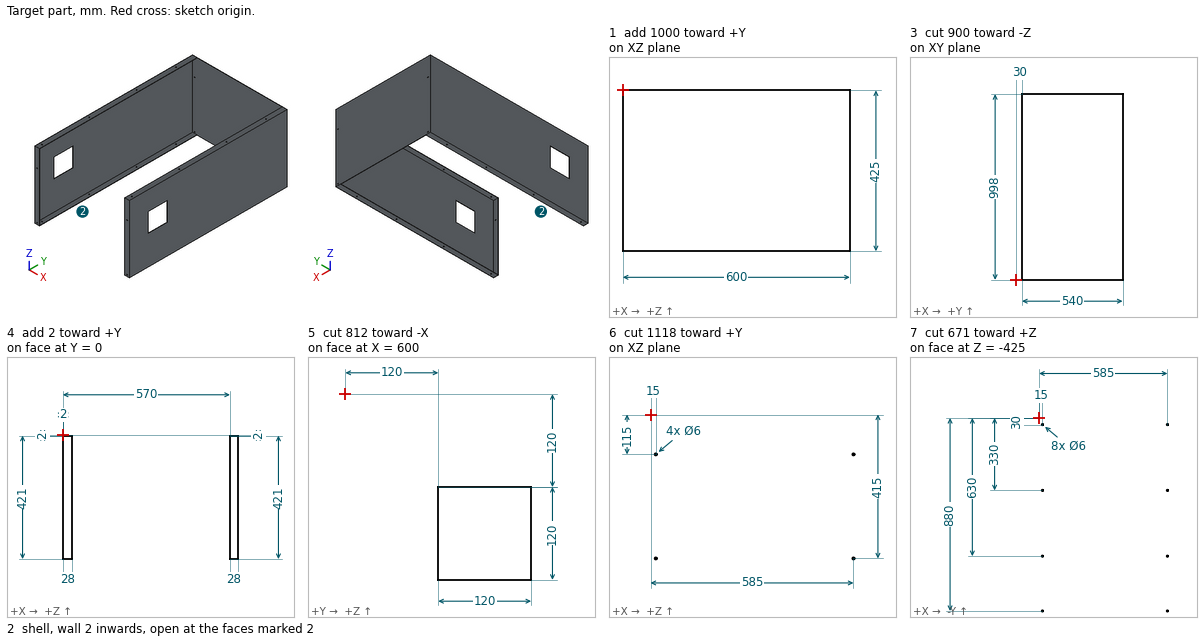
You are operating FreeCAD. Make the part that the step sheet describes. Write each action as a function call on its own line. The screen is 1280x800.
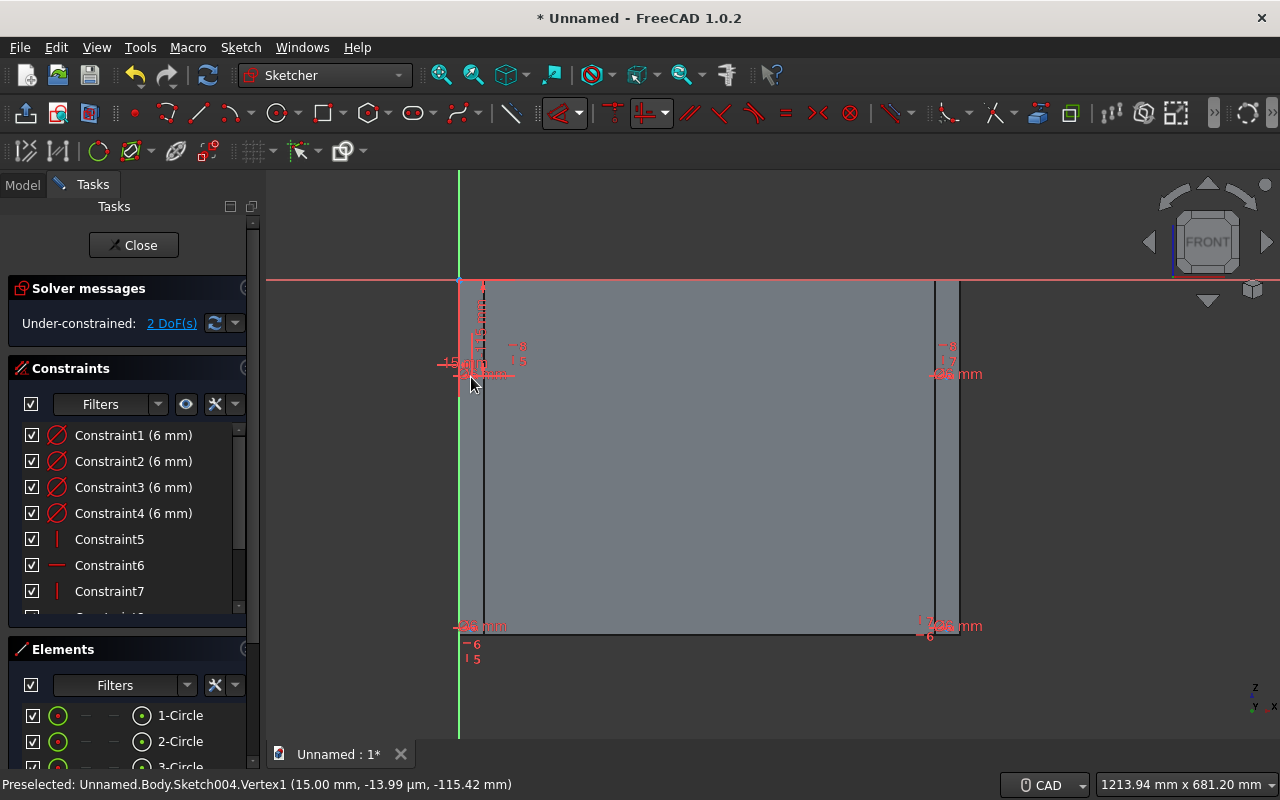
click(947, 628)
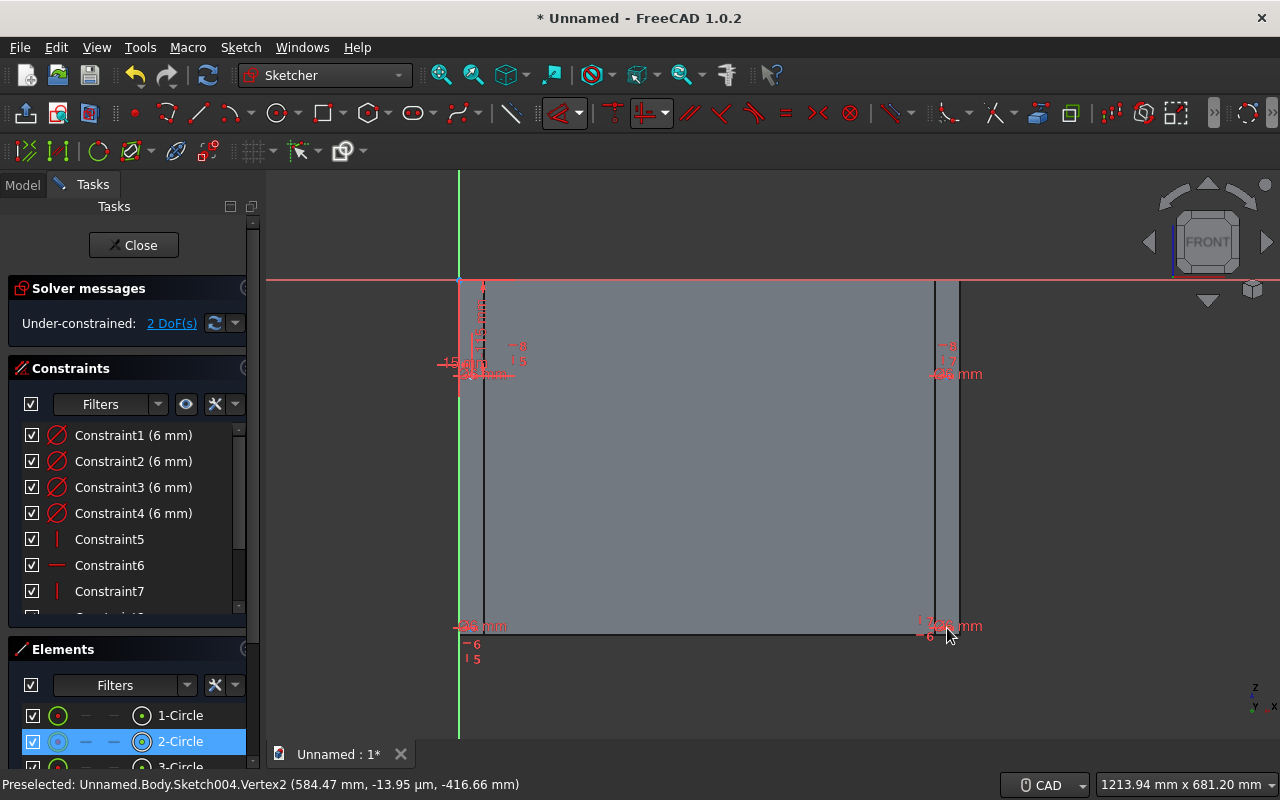
click(582, 114)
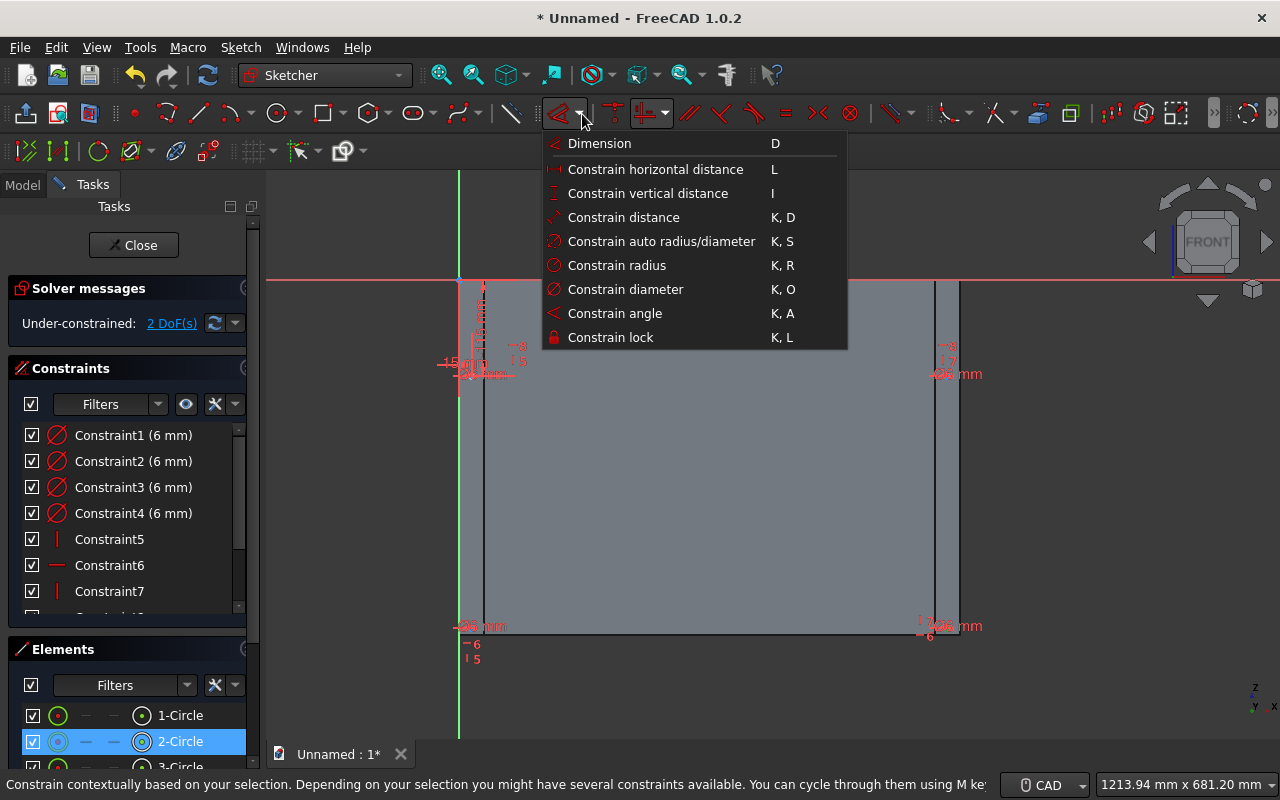
click(695, 169)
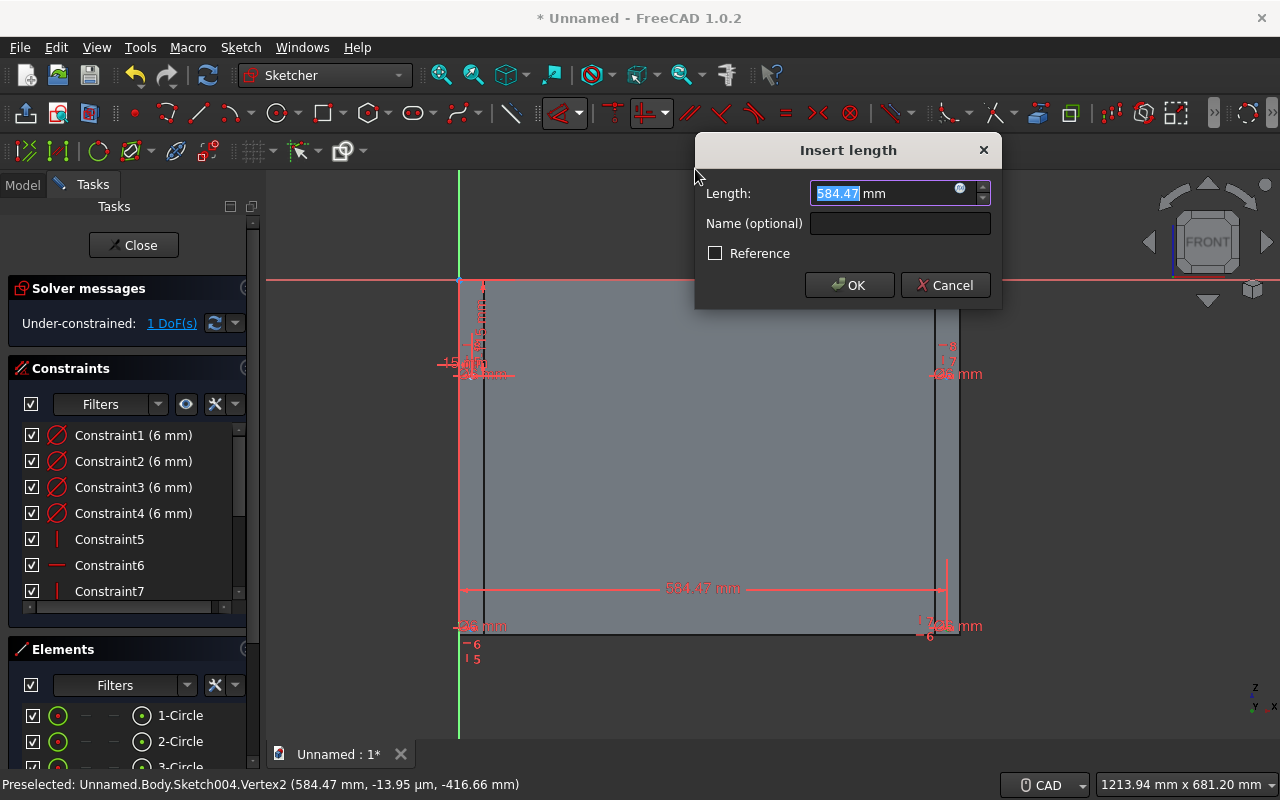
text(585)
key(Return)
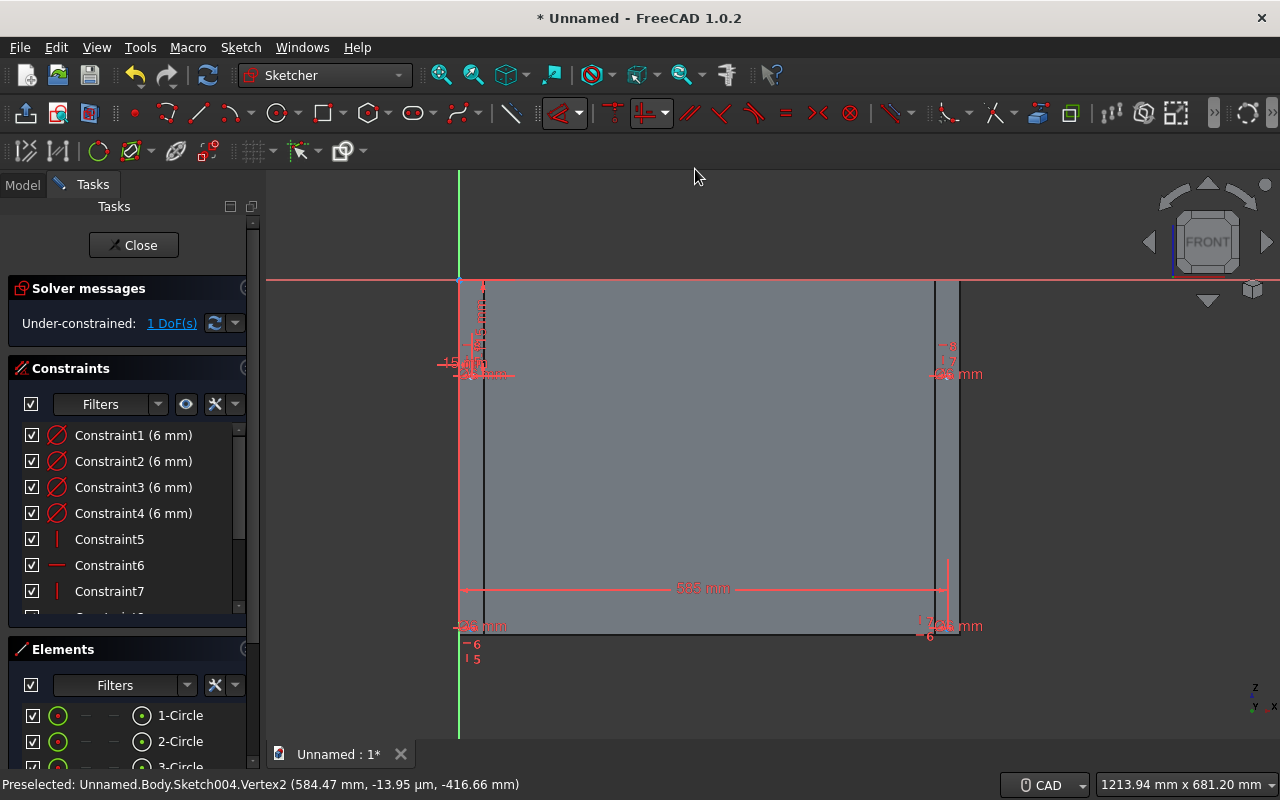
click(948, 628)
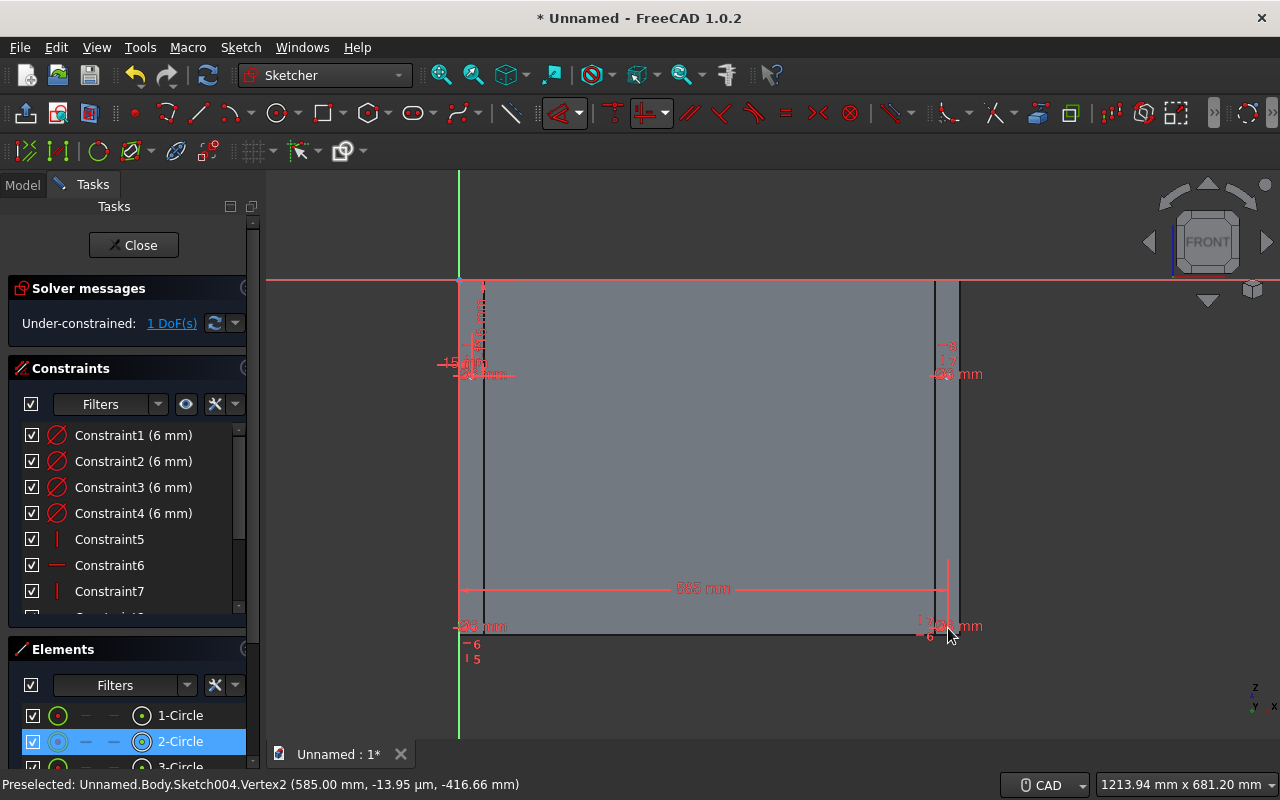
click(582, 114)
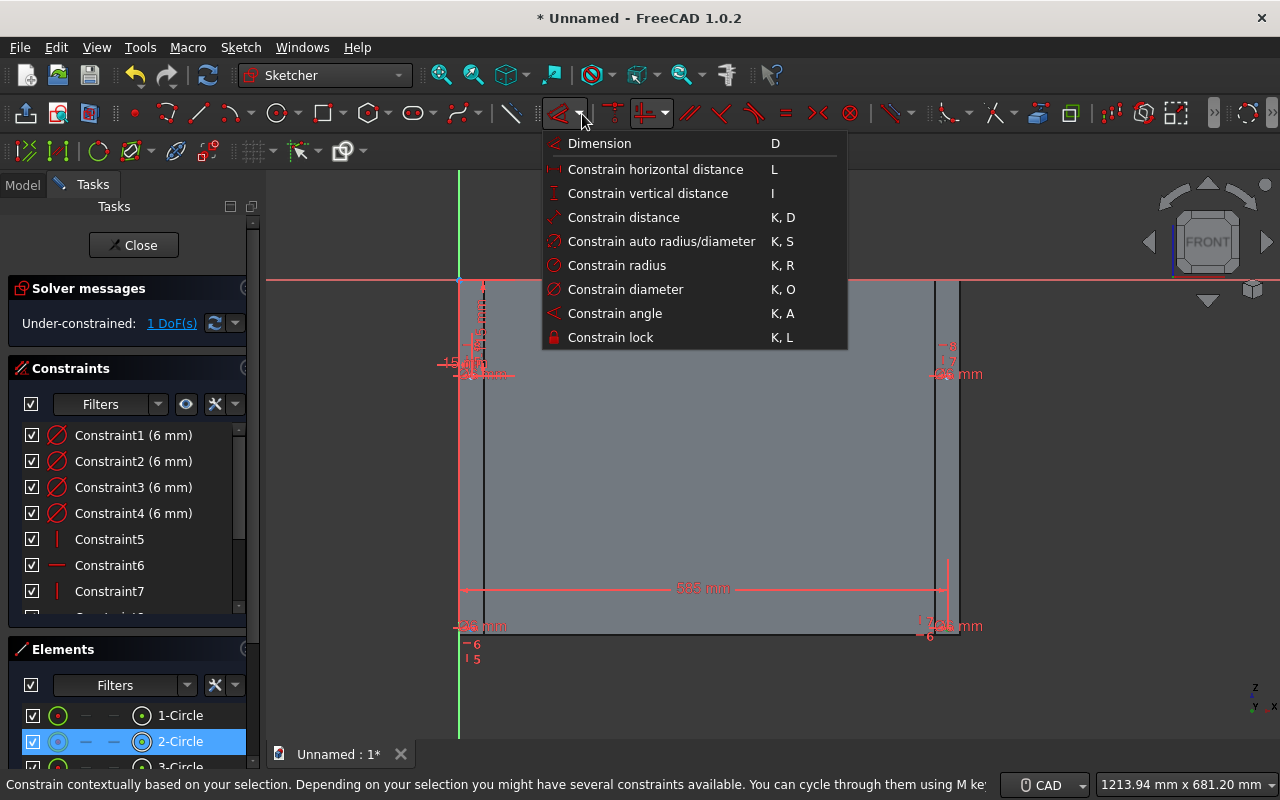
click(695, 193)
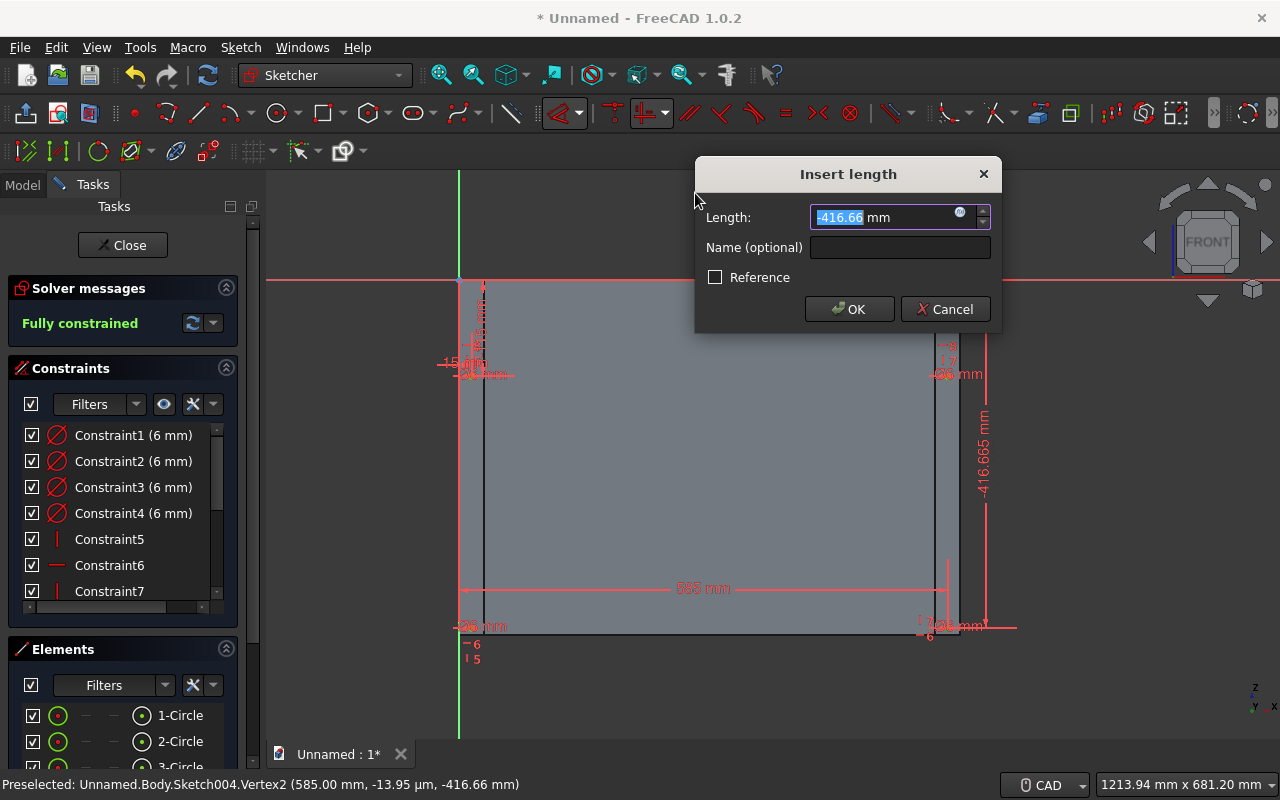
text(-415)
key(Return)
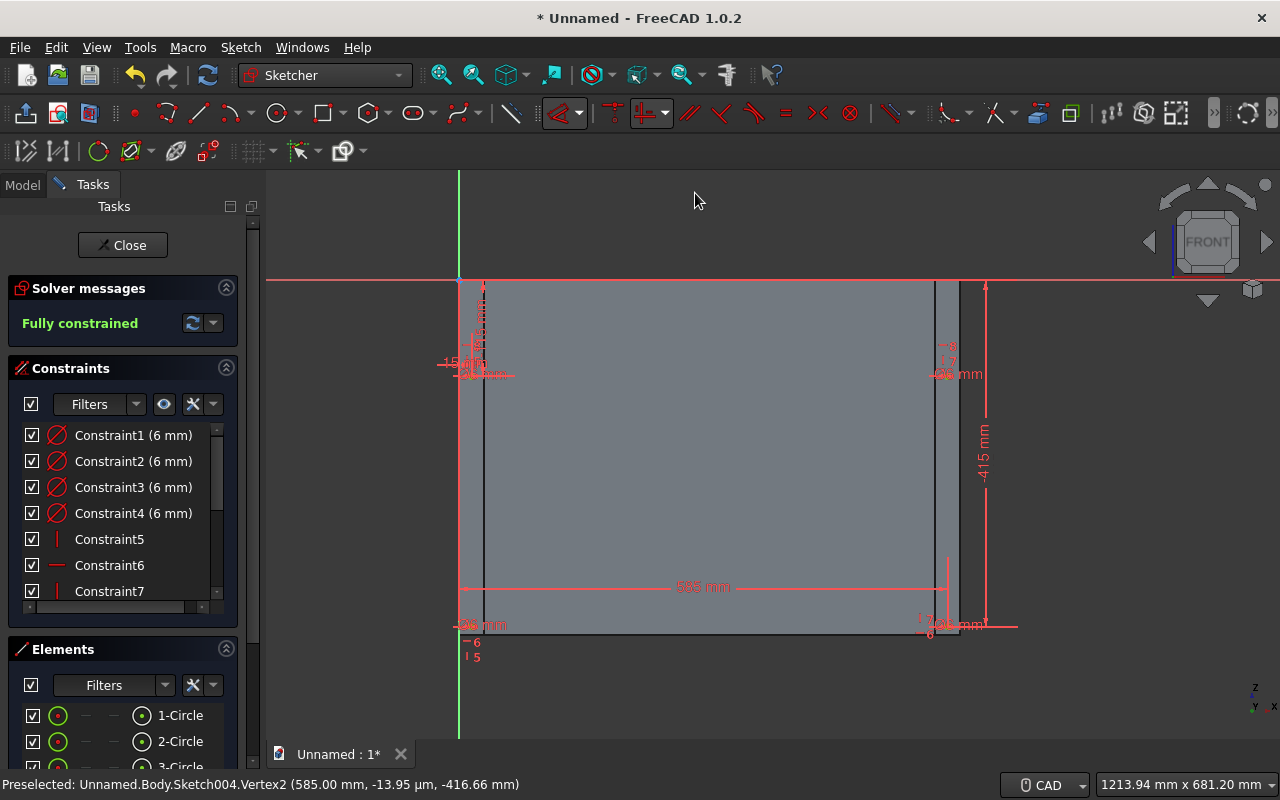
click(123, 245)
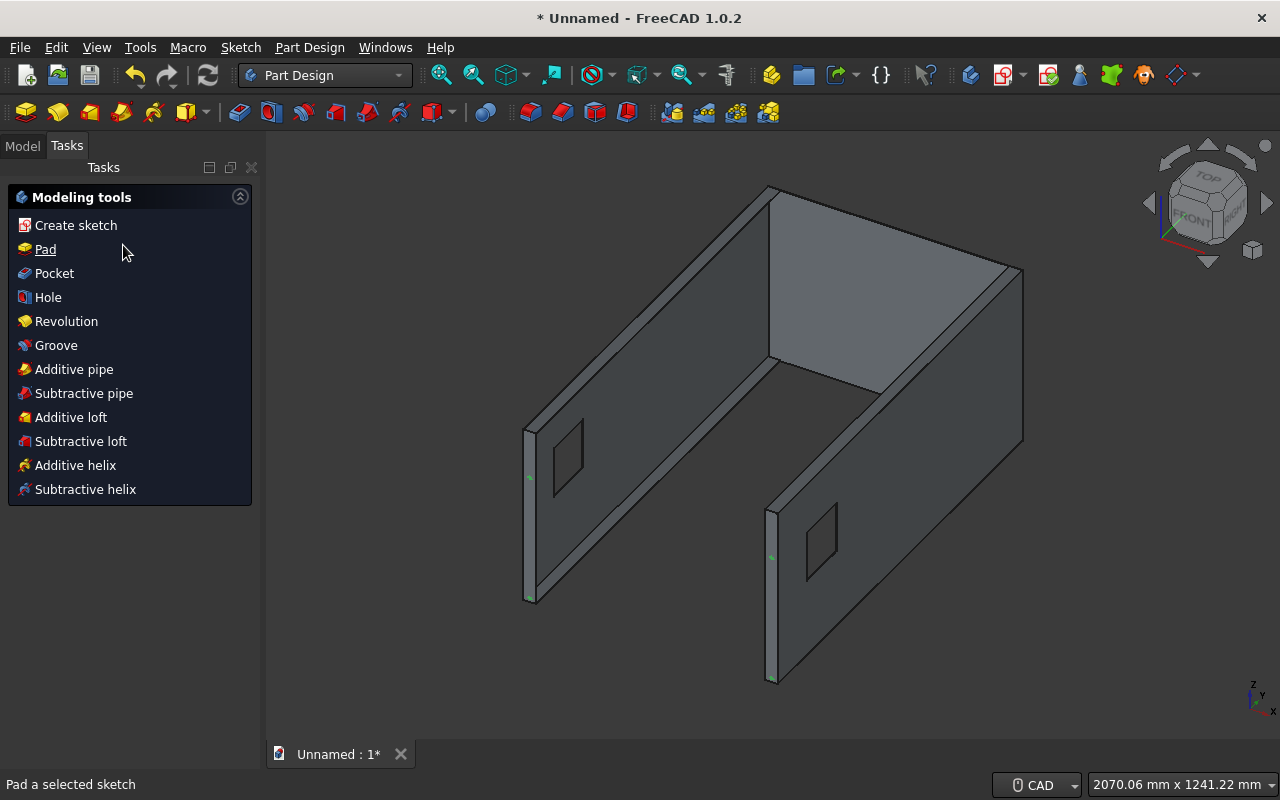
click(240, 112)